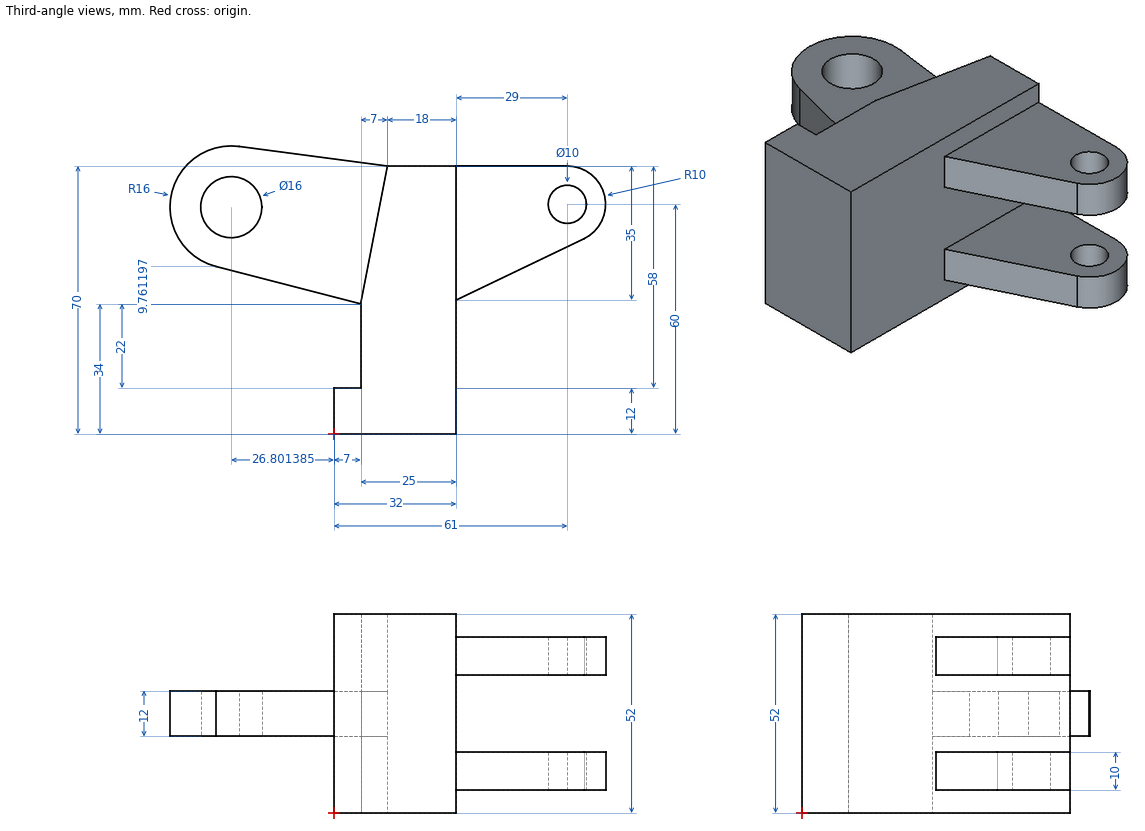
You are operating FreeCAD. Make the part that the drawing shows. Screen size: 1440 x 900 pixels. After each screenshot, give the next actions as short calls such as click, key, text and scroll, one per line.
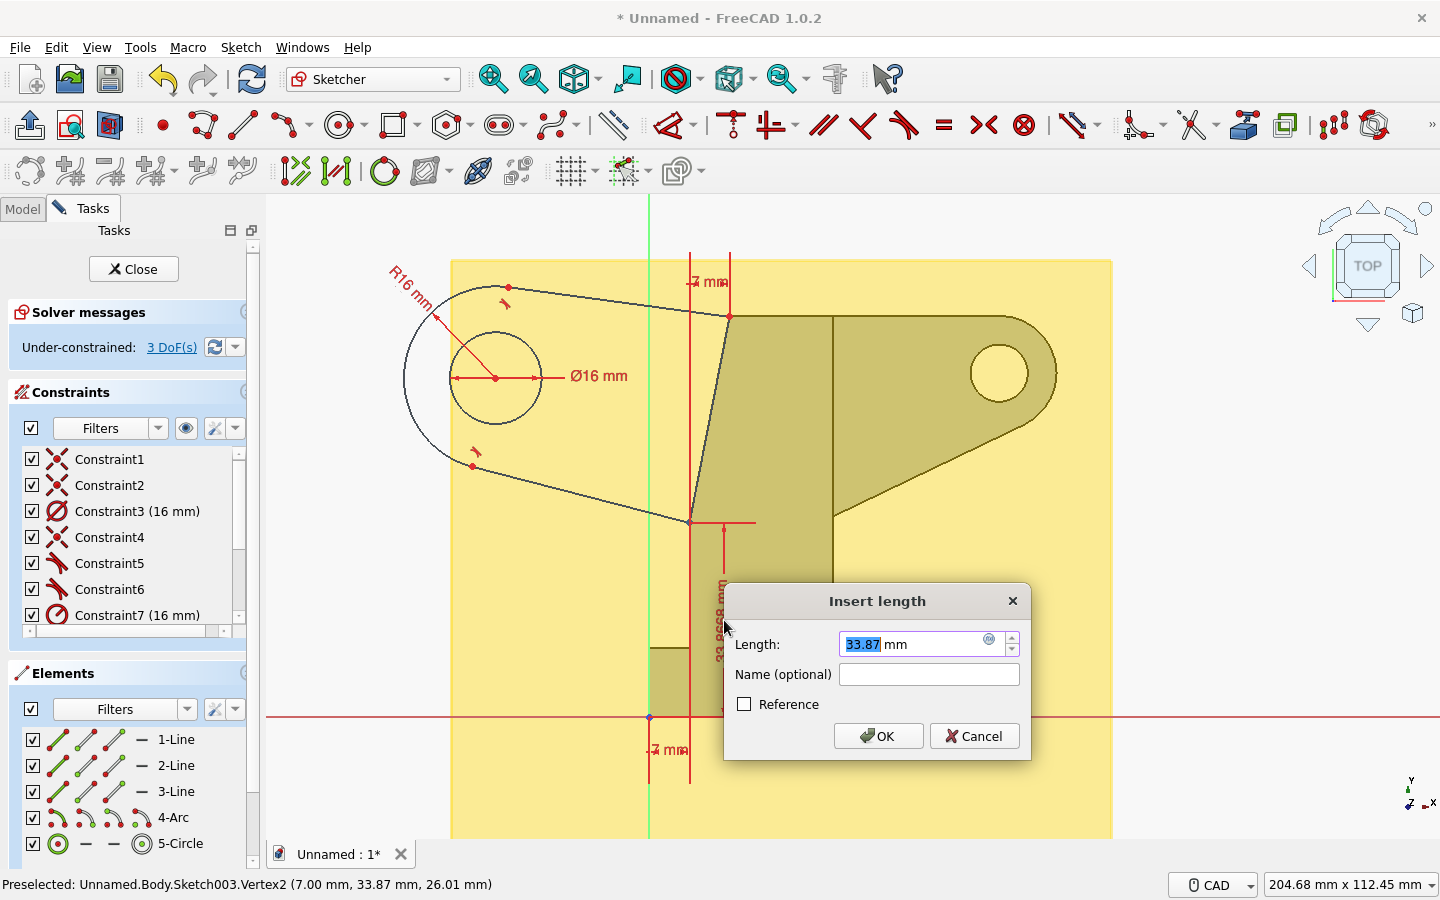
text(34)
key(Return)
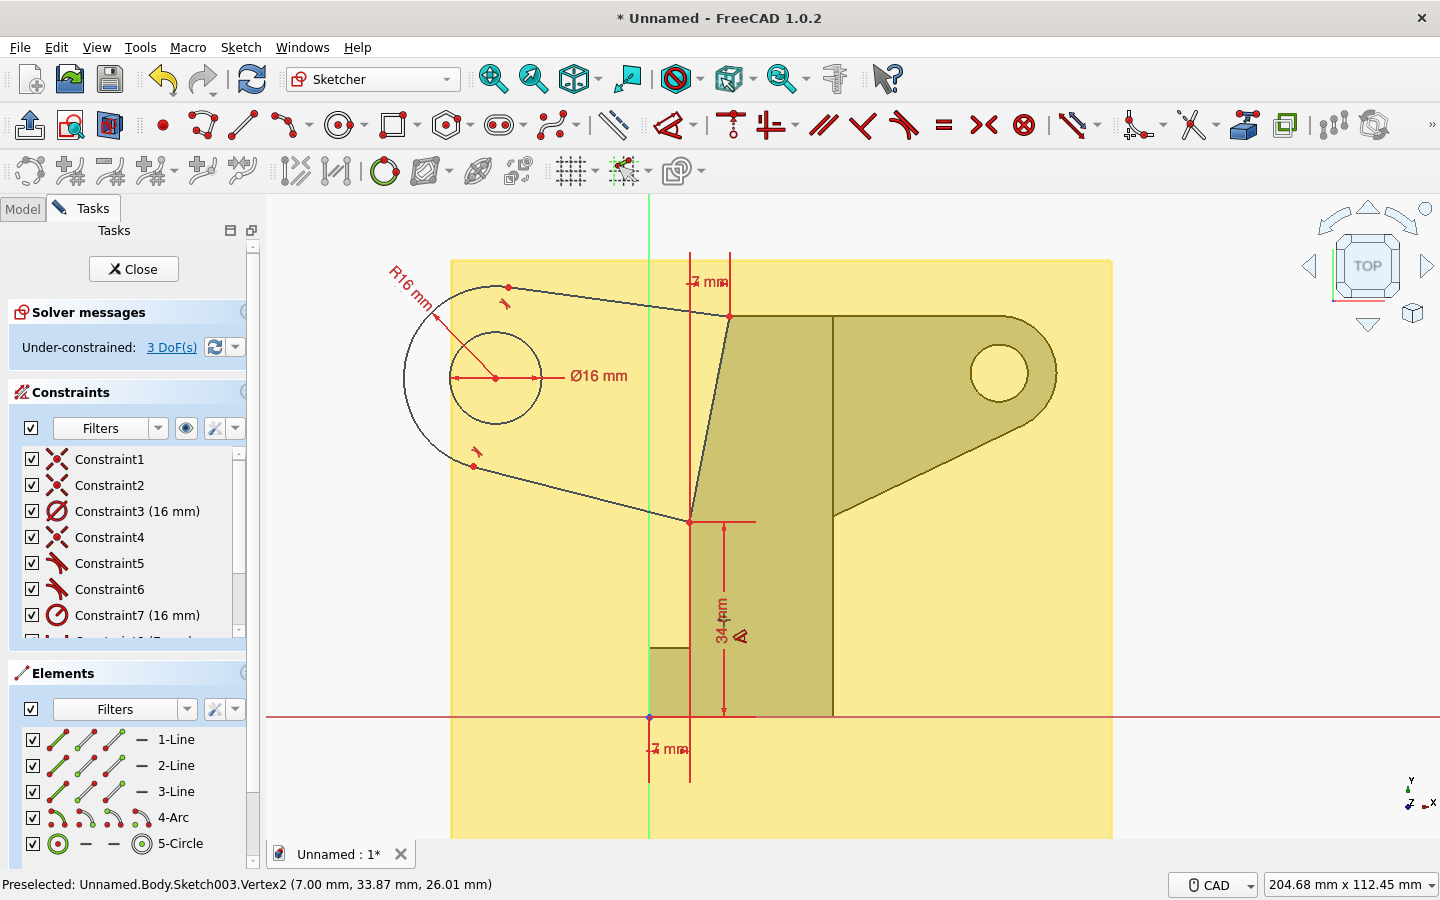
click(730, 317)
click(764, 517)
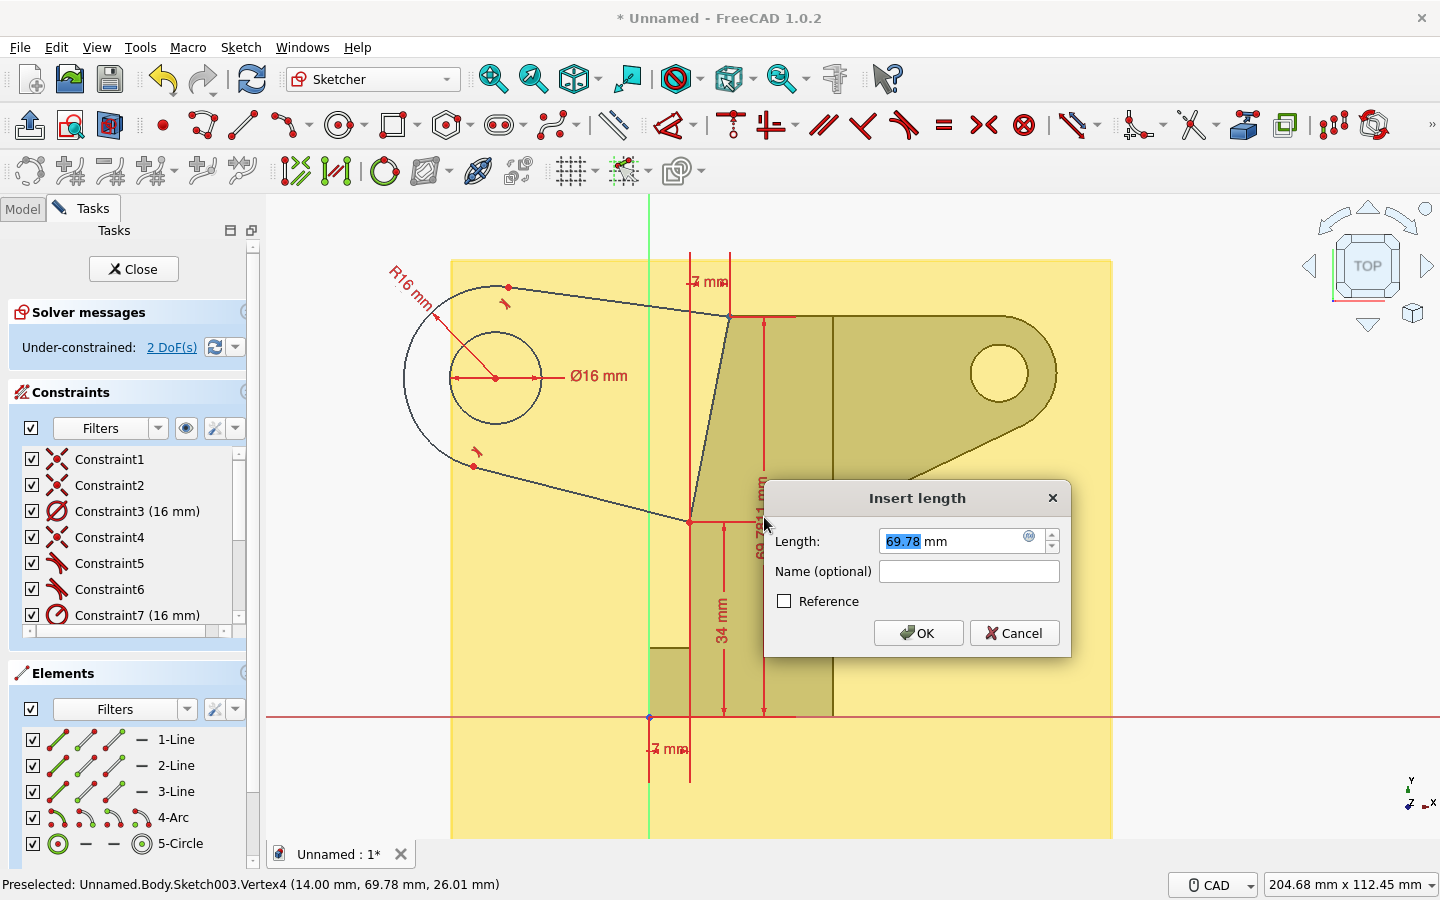
text(70)
key(Return)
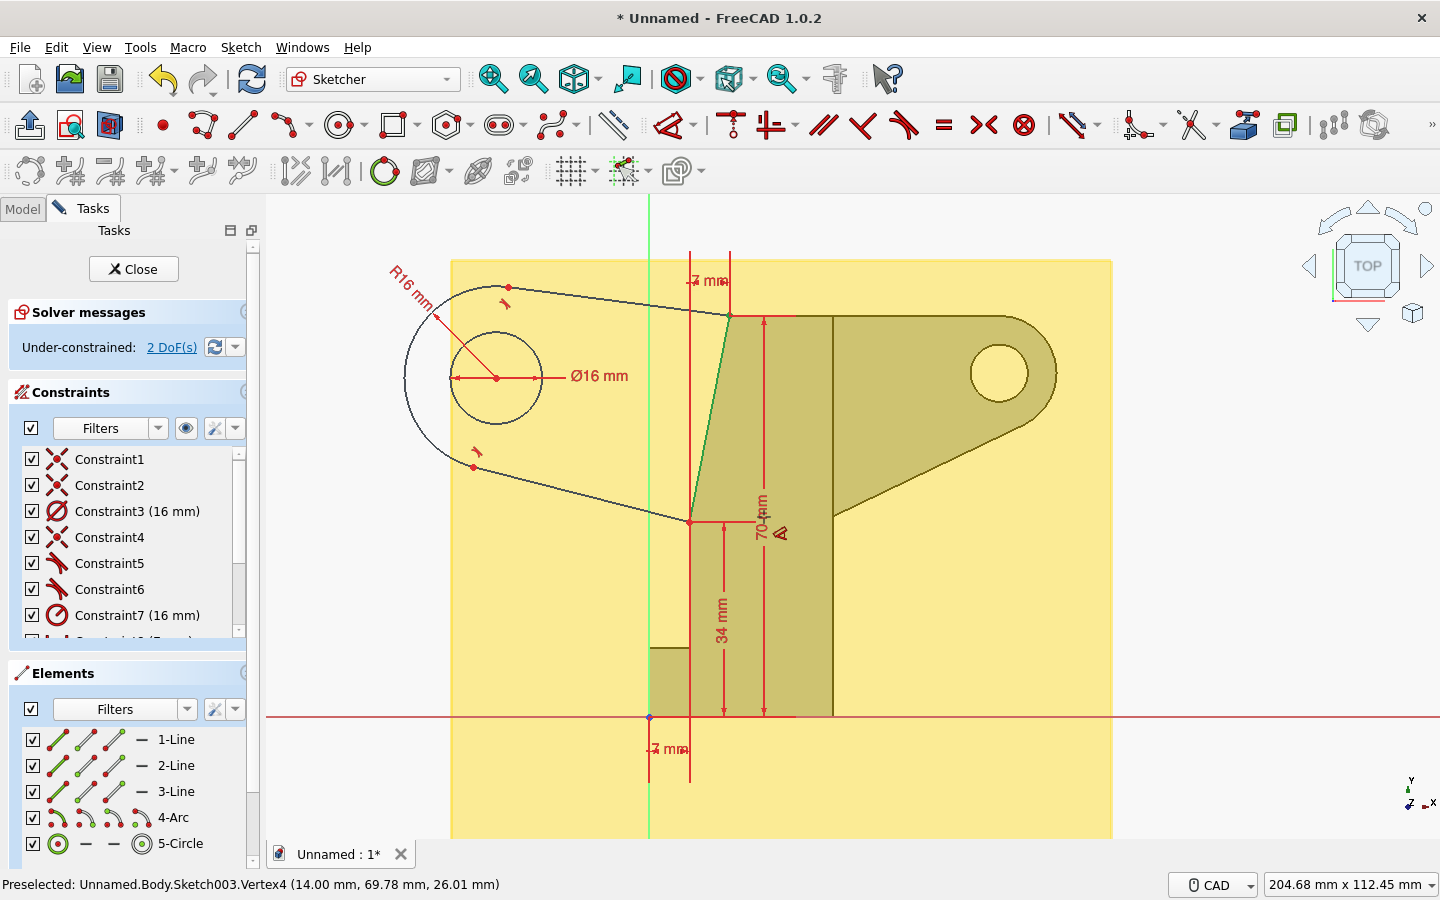
click(538, 484)
click(724, 495)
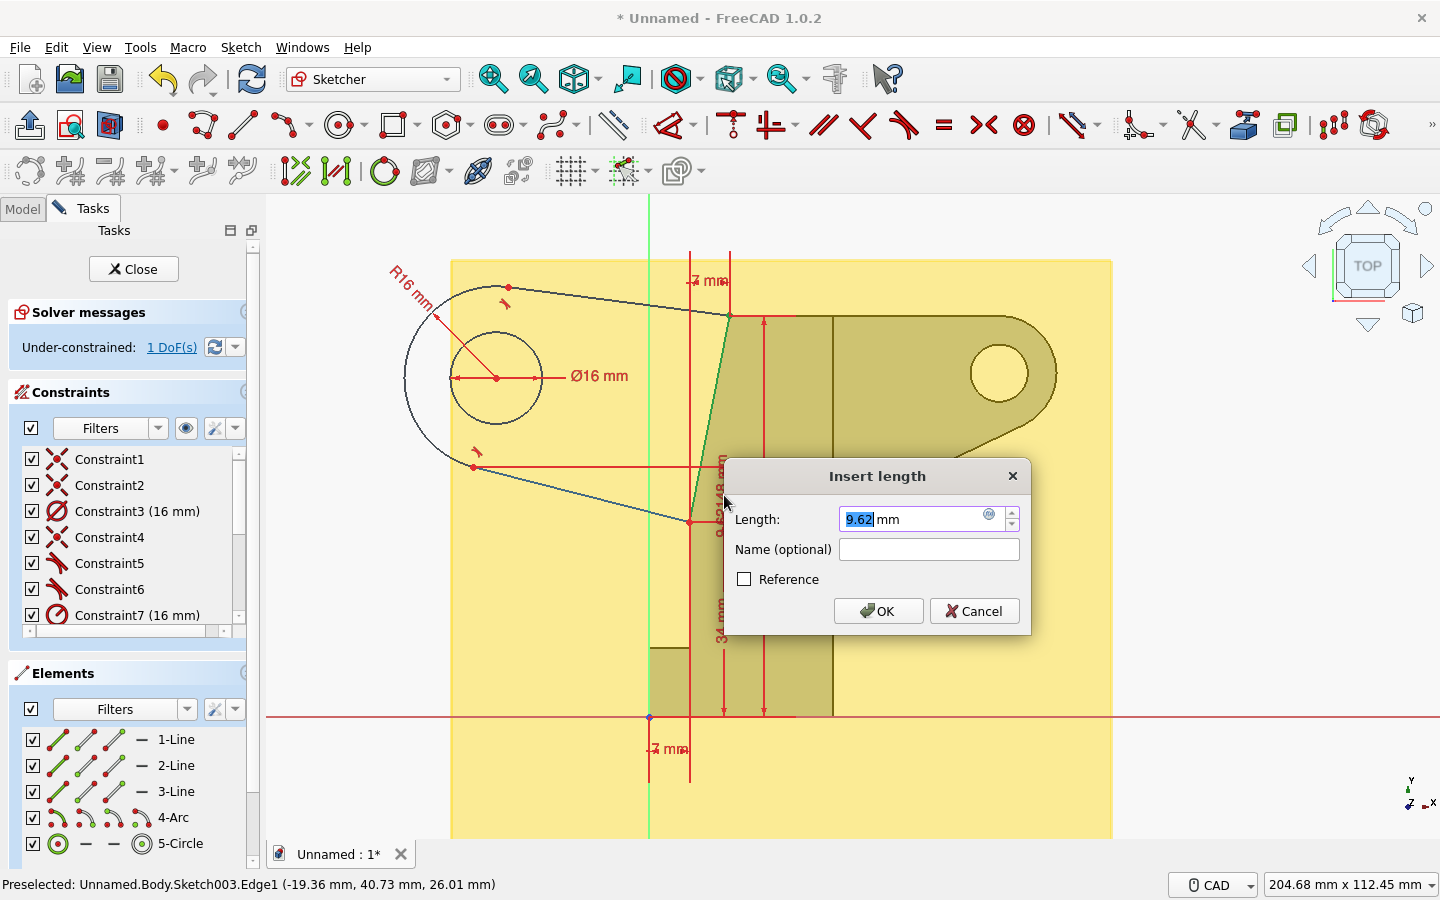
text(9.761197)
key(Return)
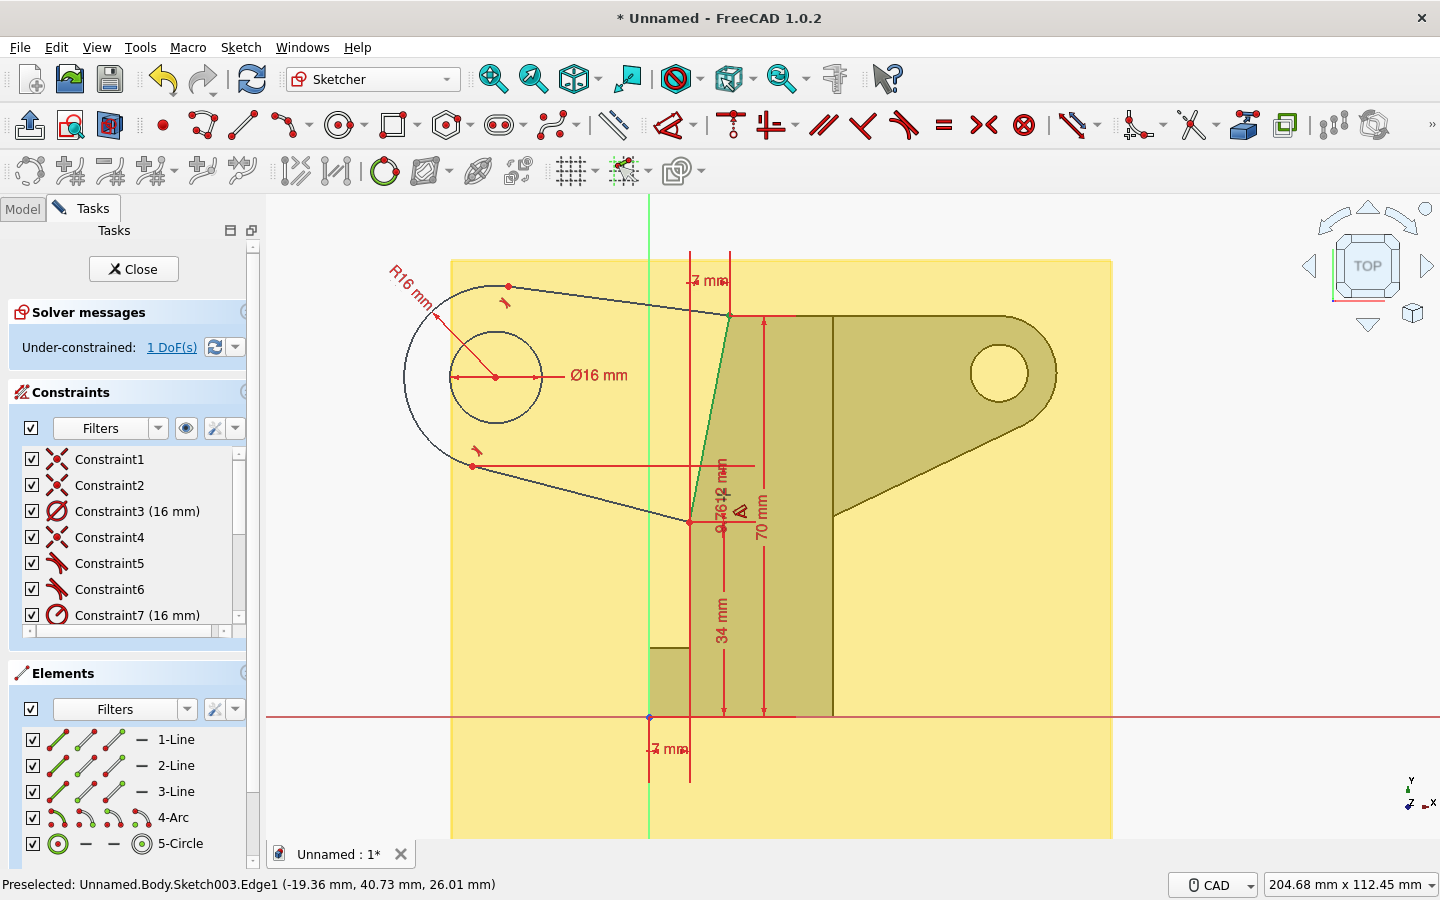
click(496, 377)
click(573, 751)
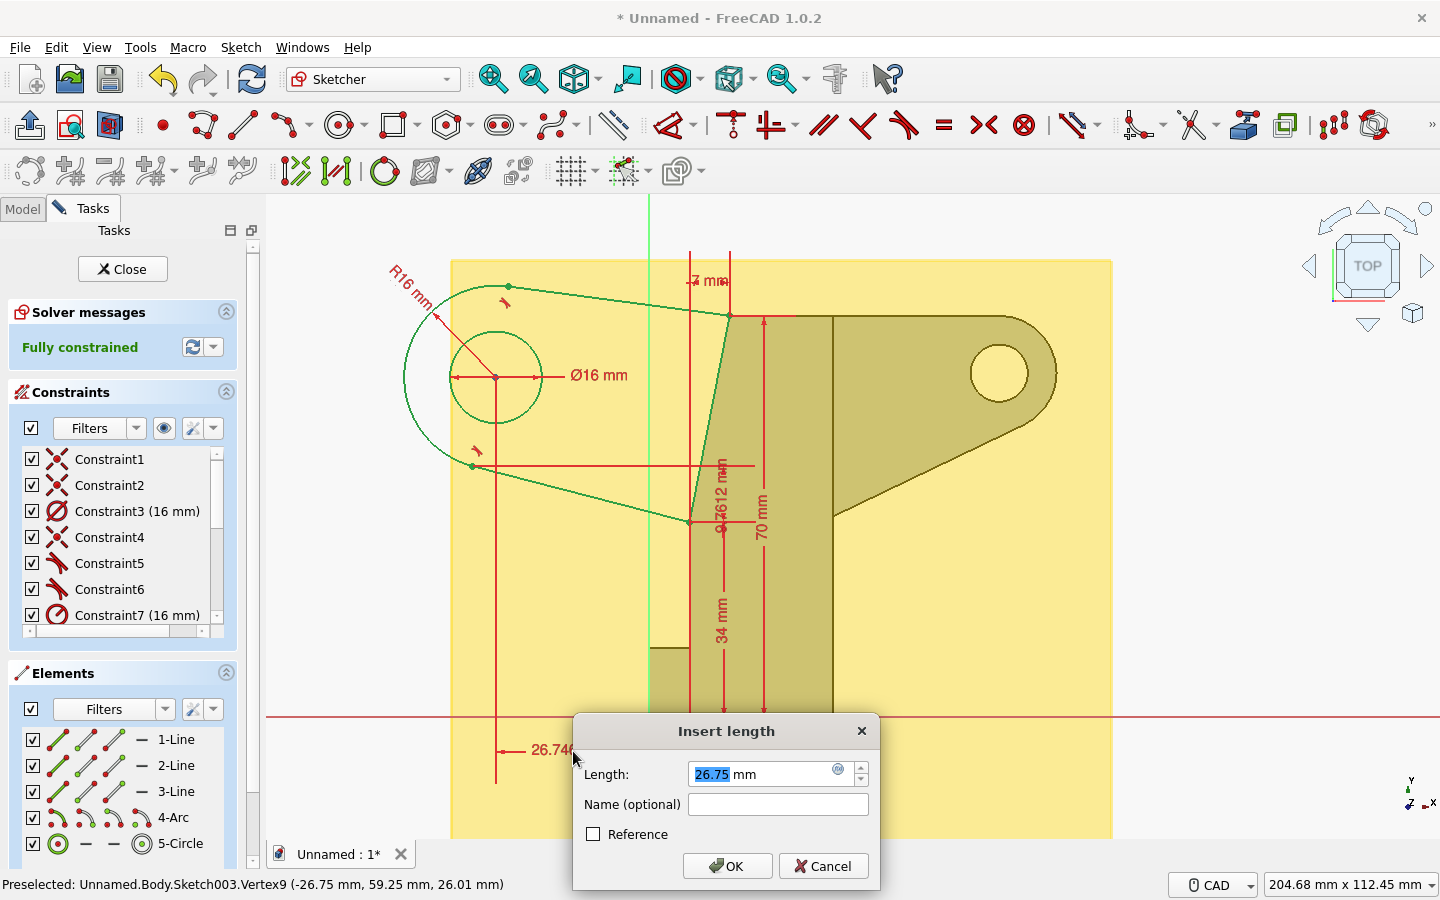
text(26.801385)
key(Return)
key(Escape)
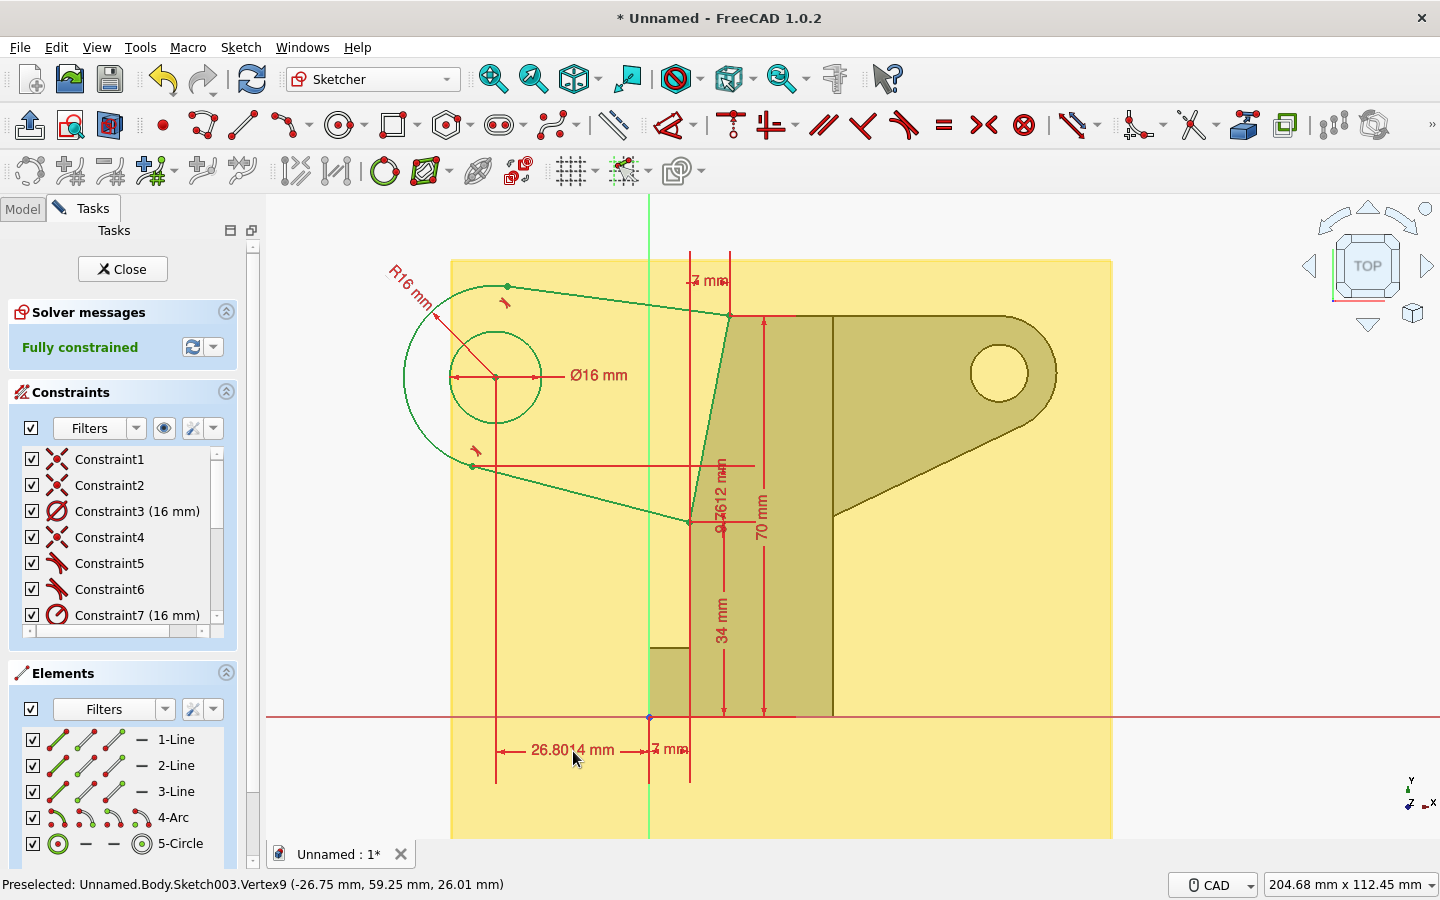
click(123, 269)